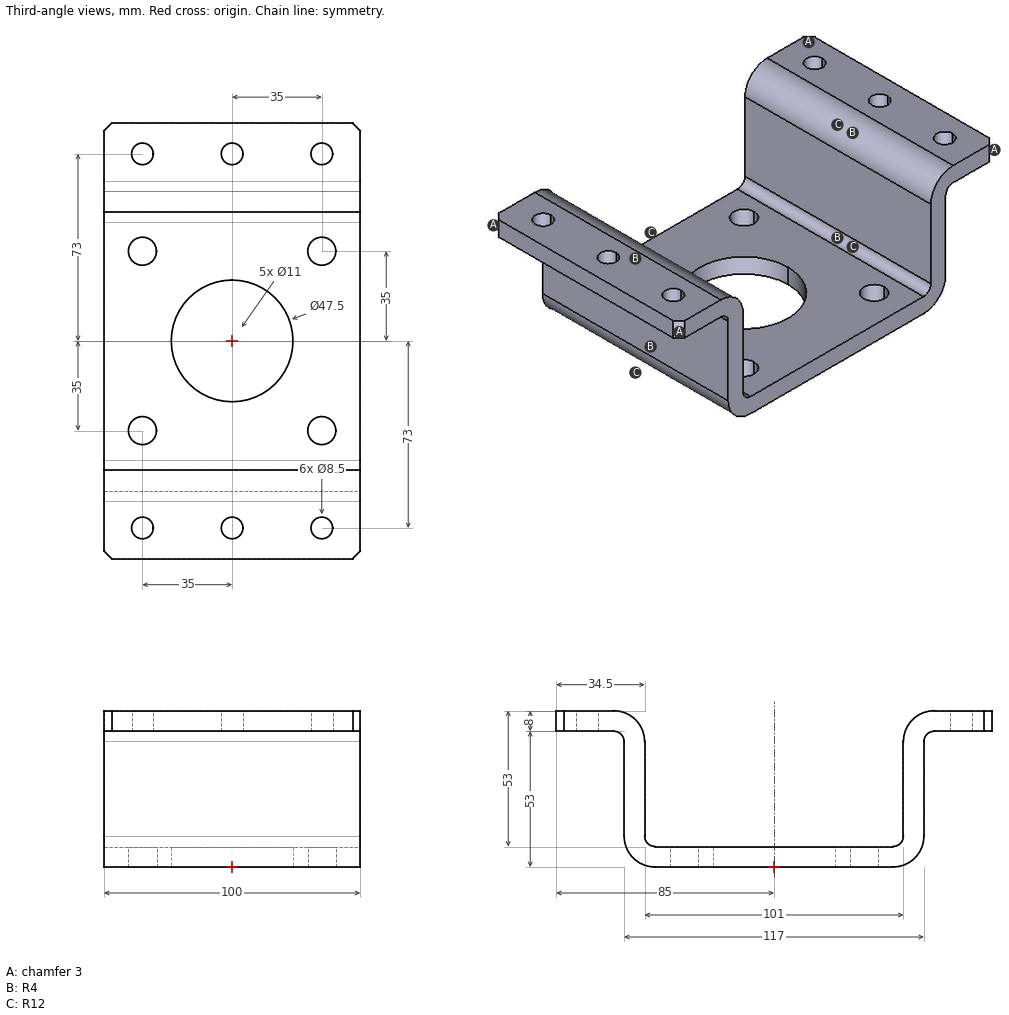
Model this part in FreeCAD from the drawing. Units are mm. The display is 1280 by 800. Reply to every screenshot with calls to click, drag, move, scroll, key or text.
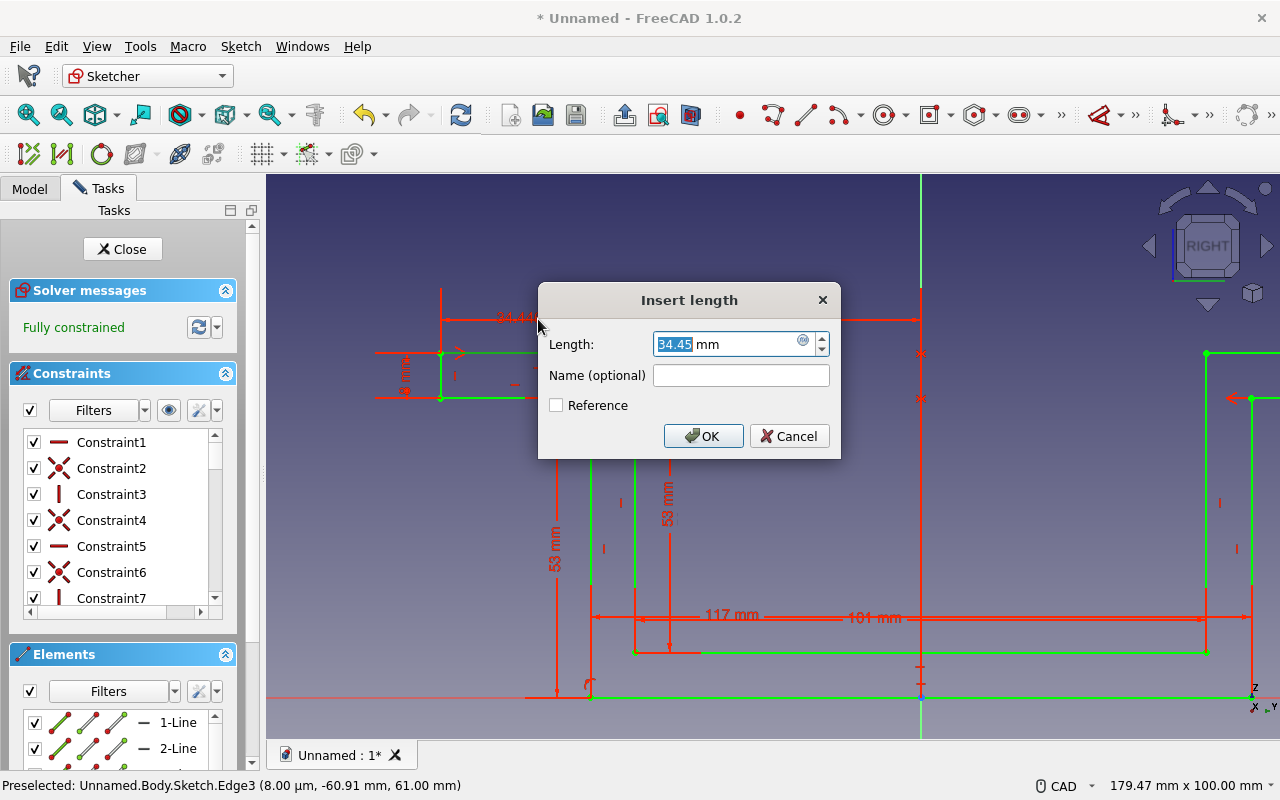
text(34.5)
key(Return)
key(Escape)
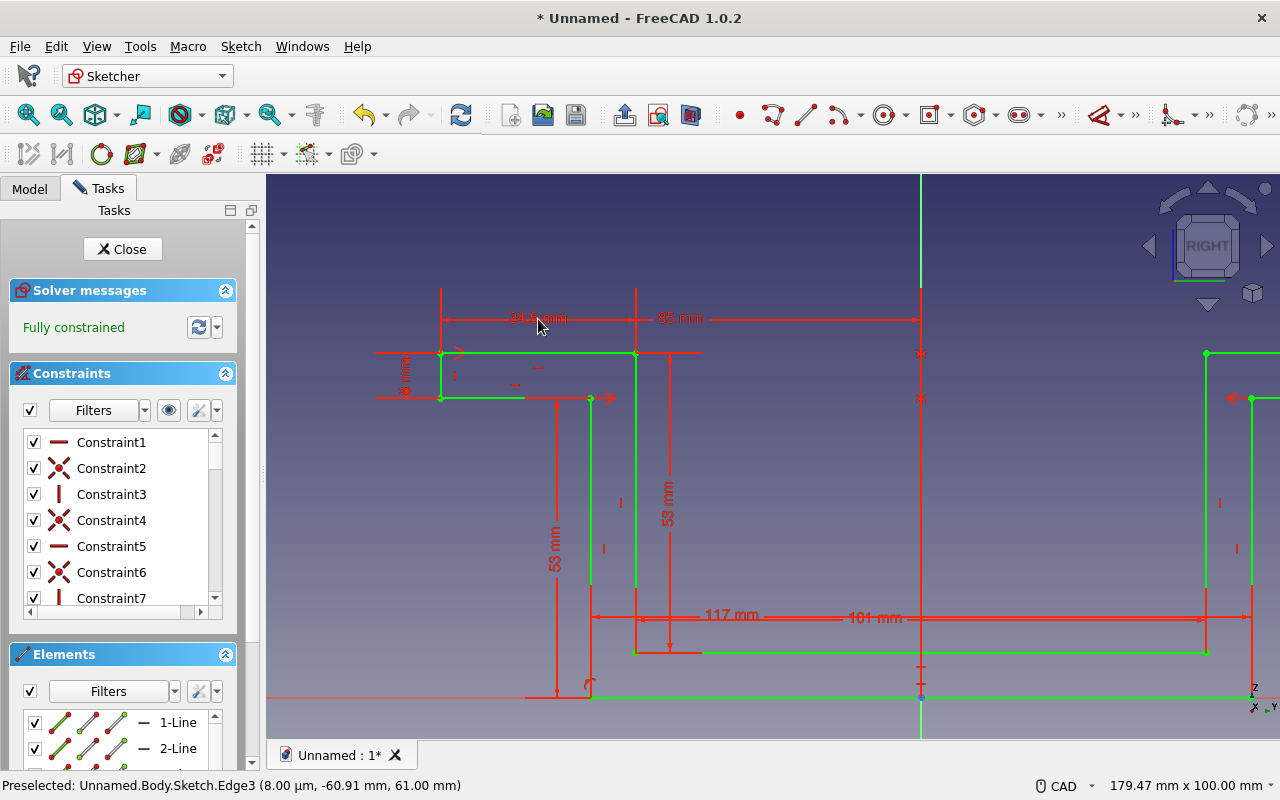
click(123, 249)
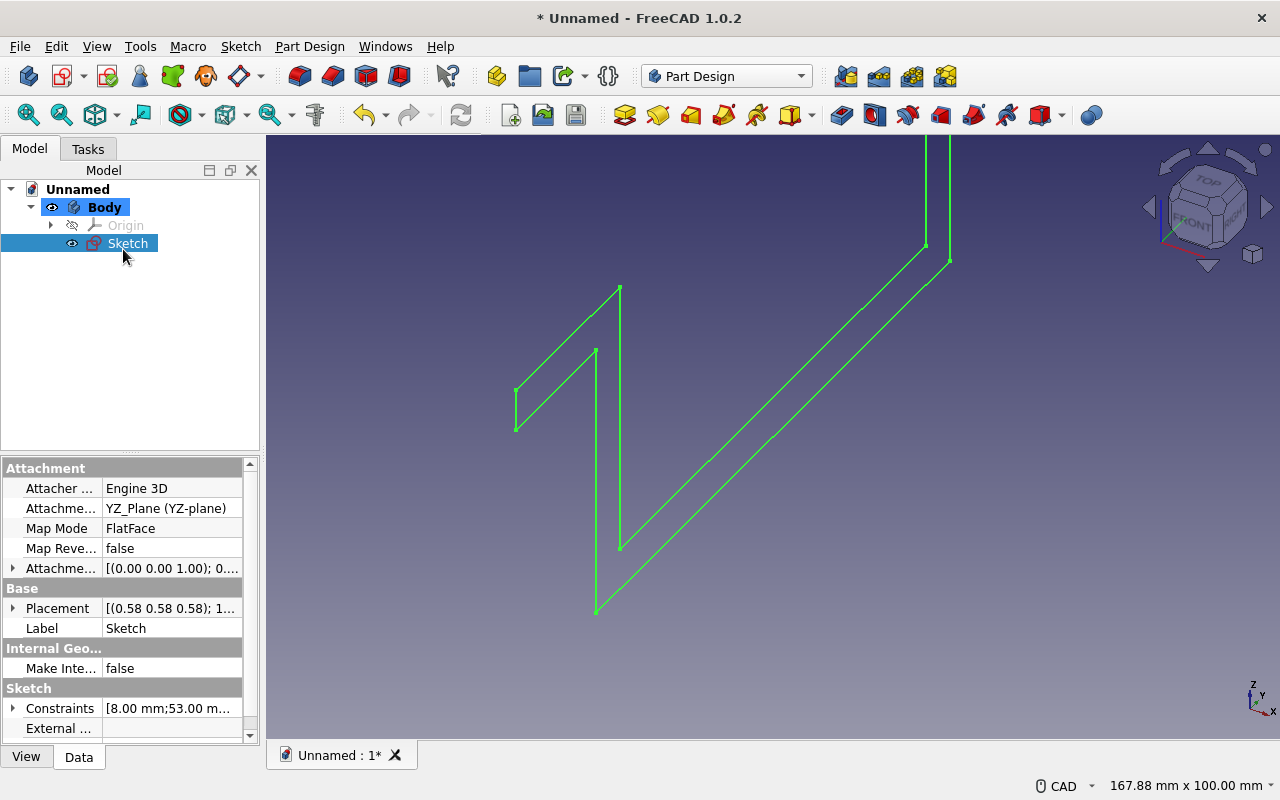
click(625, 116)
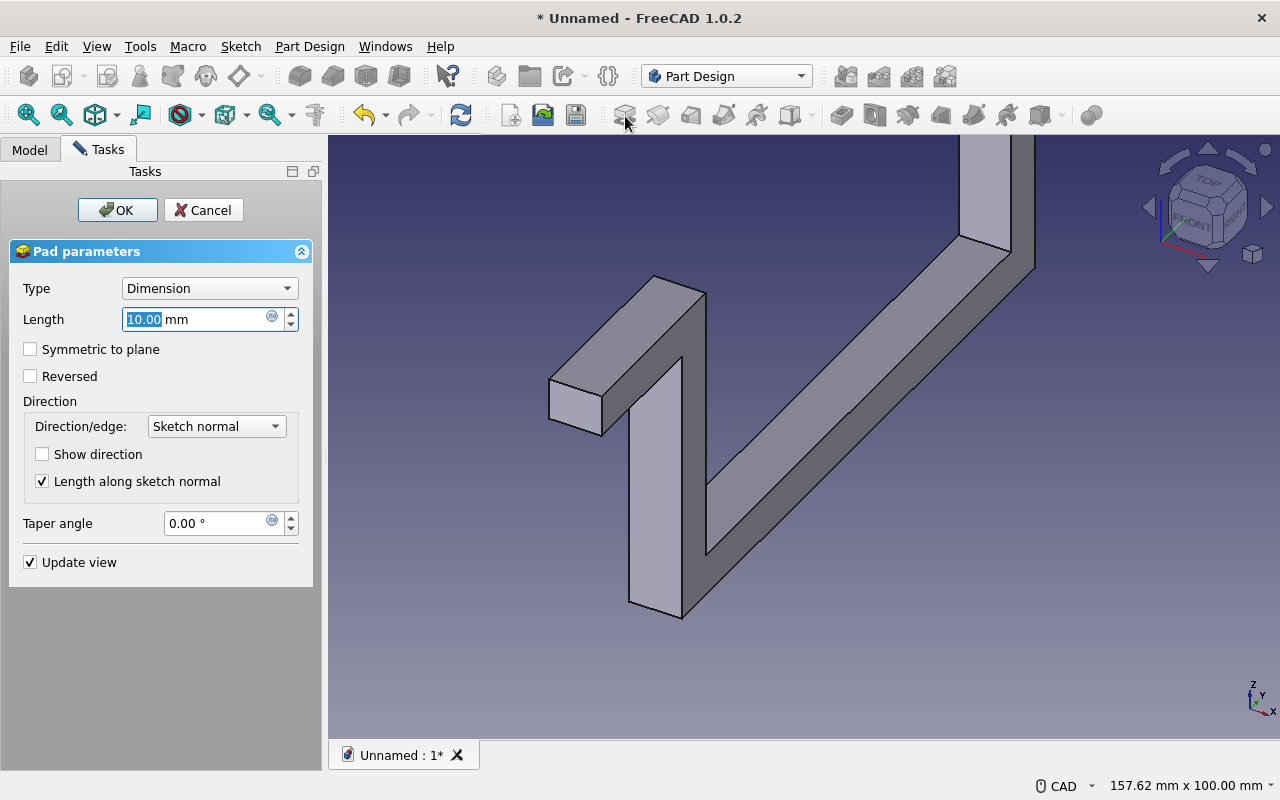
text(100)
key(Tab)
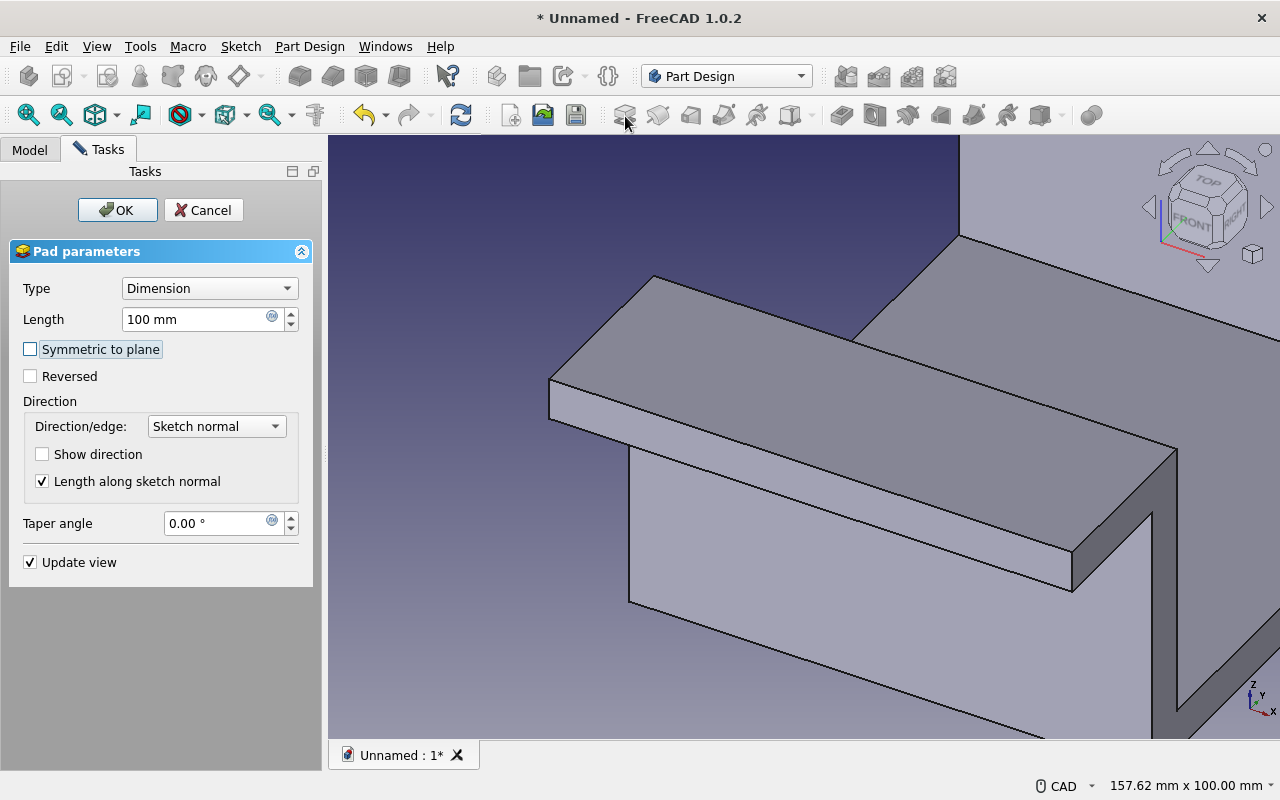
click(31, 349)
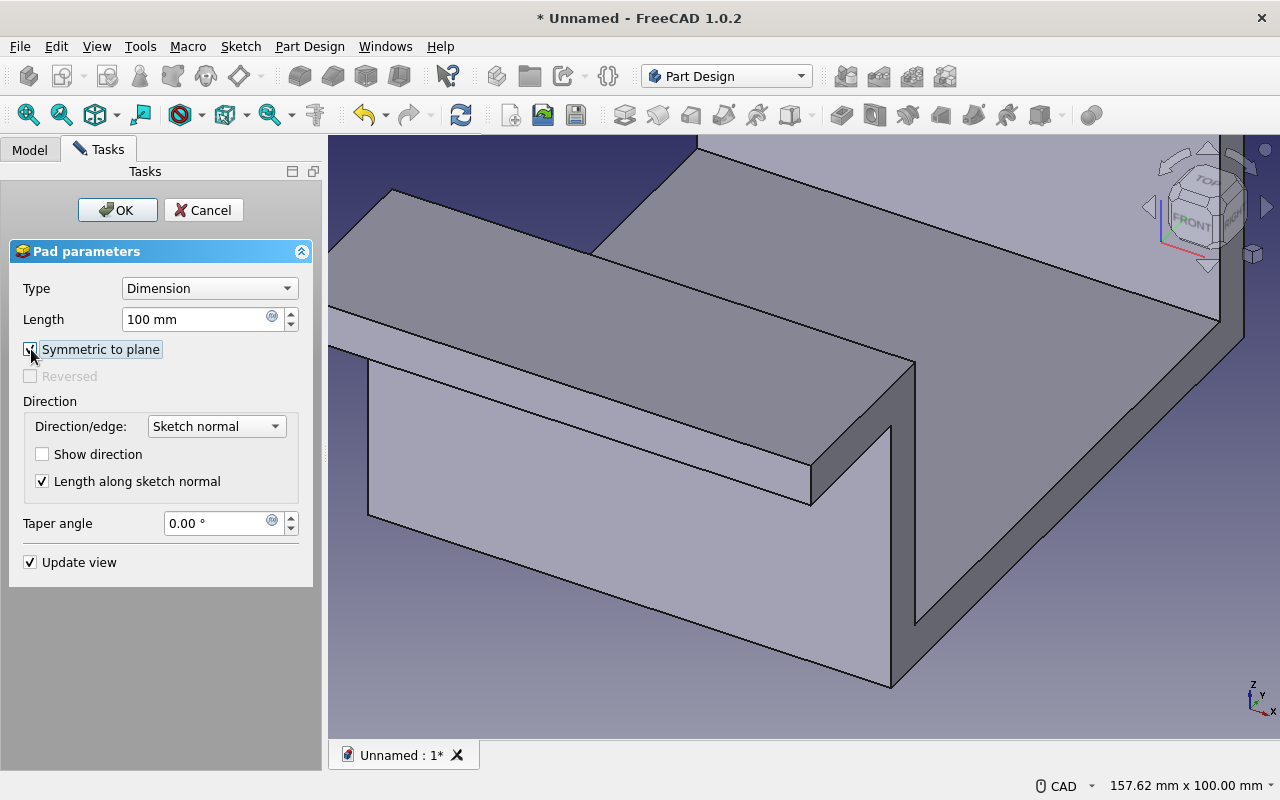
click(118, 210)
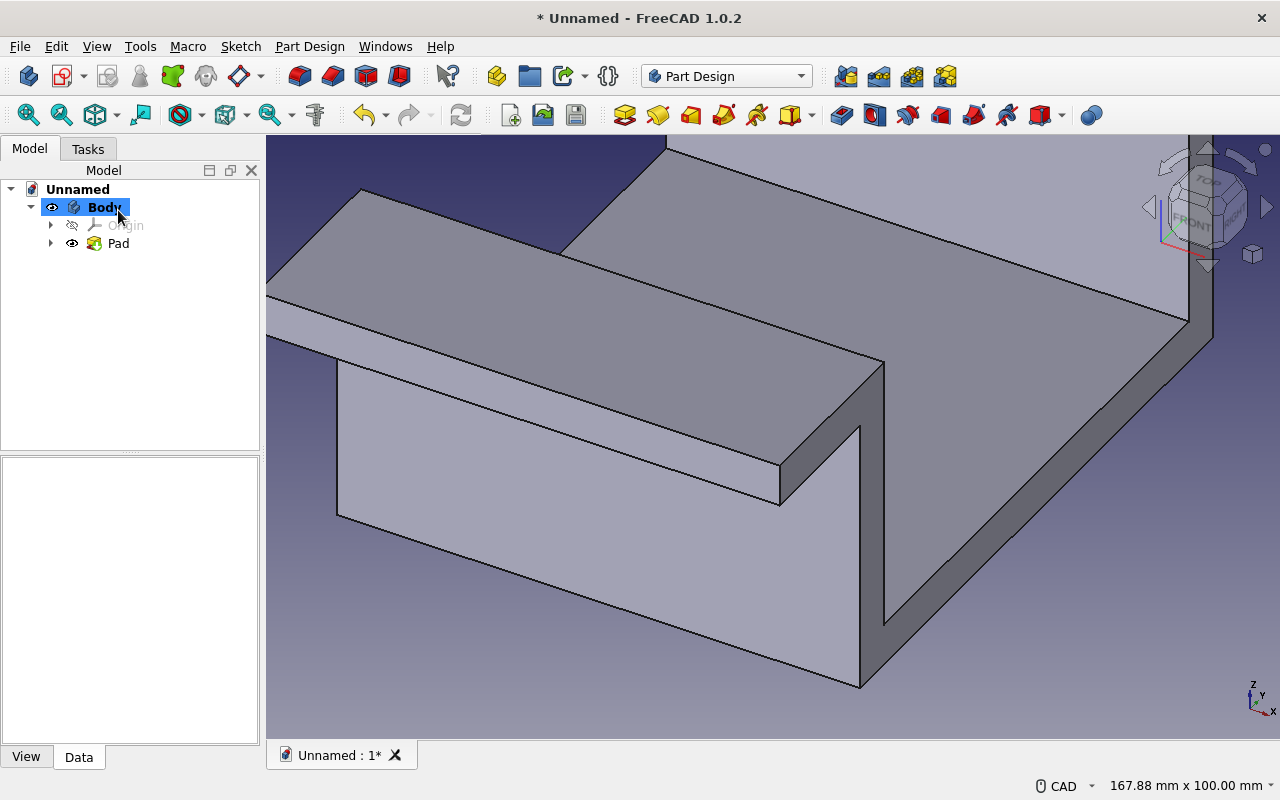
key(v)
key(f)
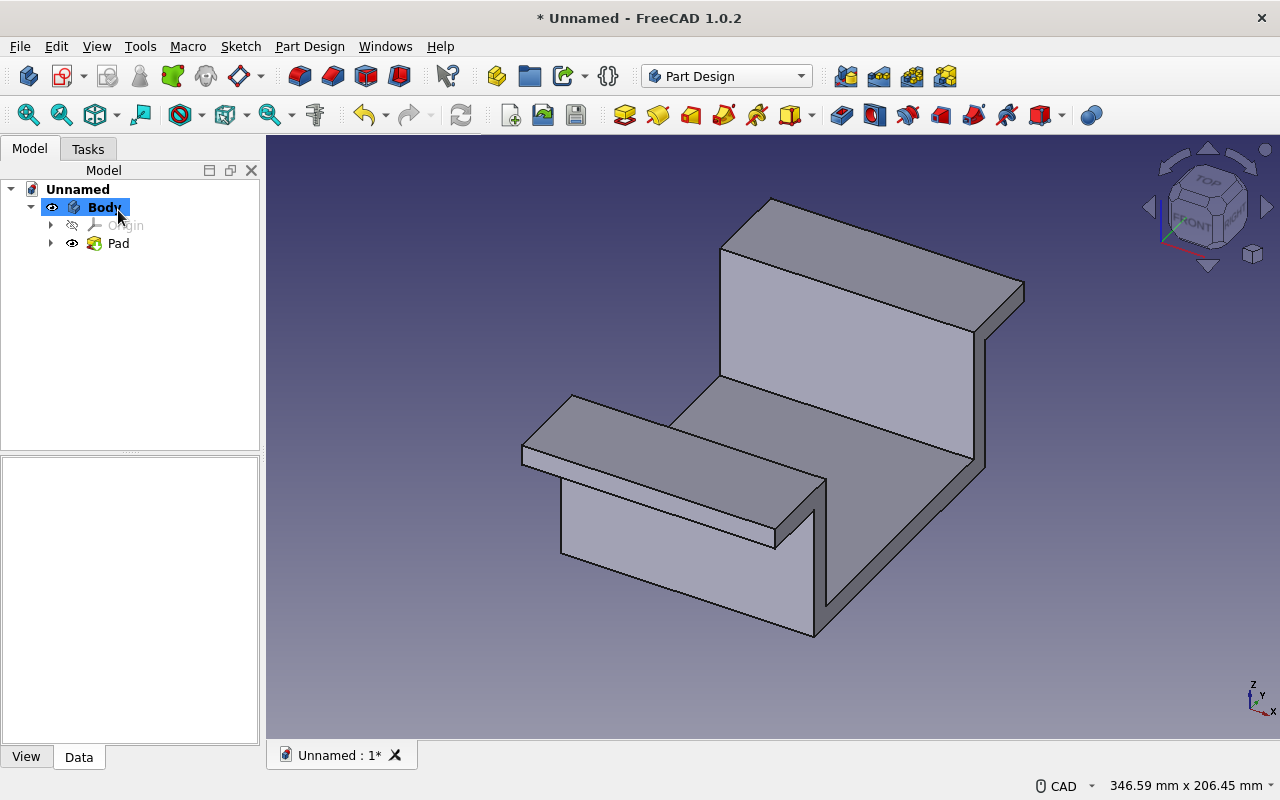
key(5)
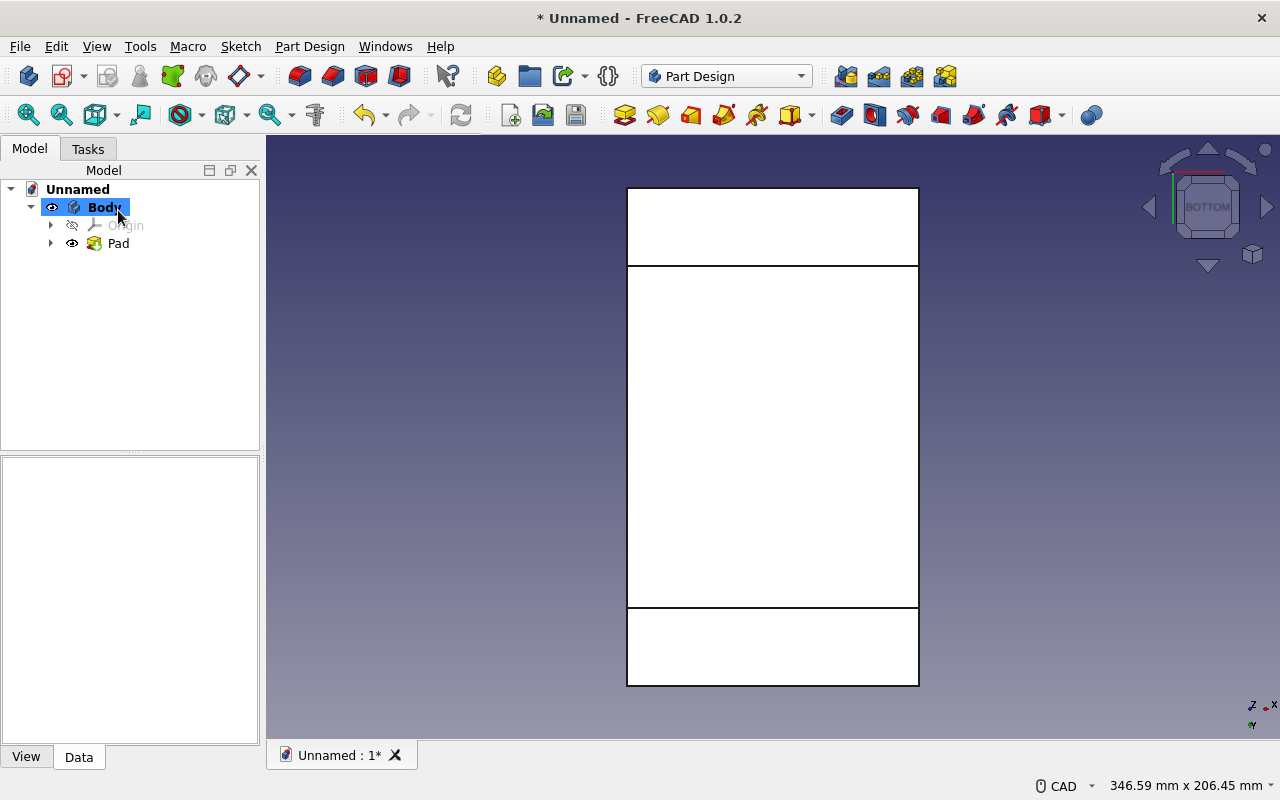
click(773, 436)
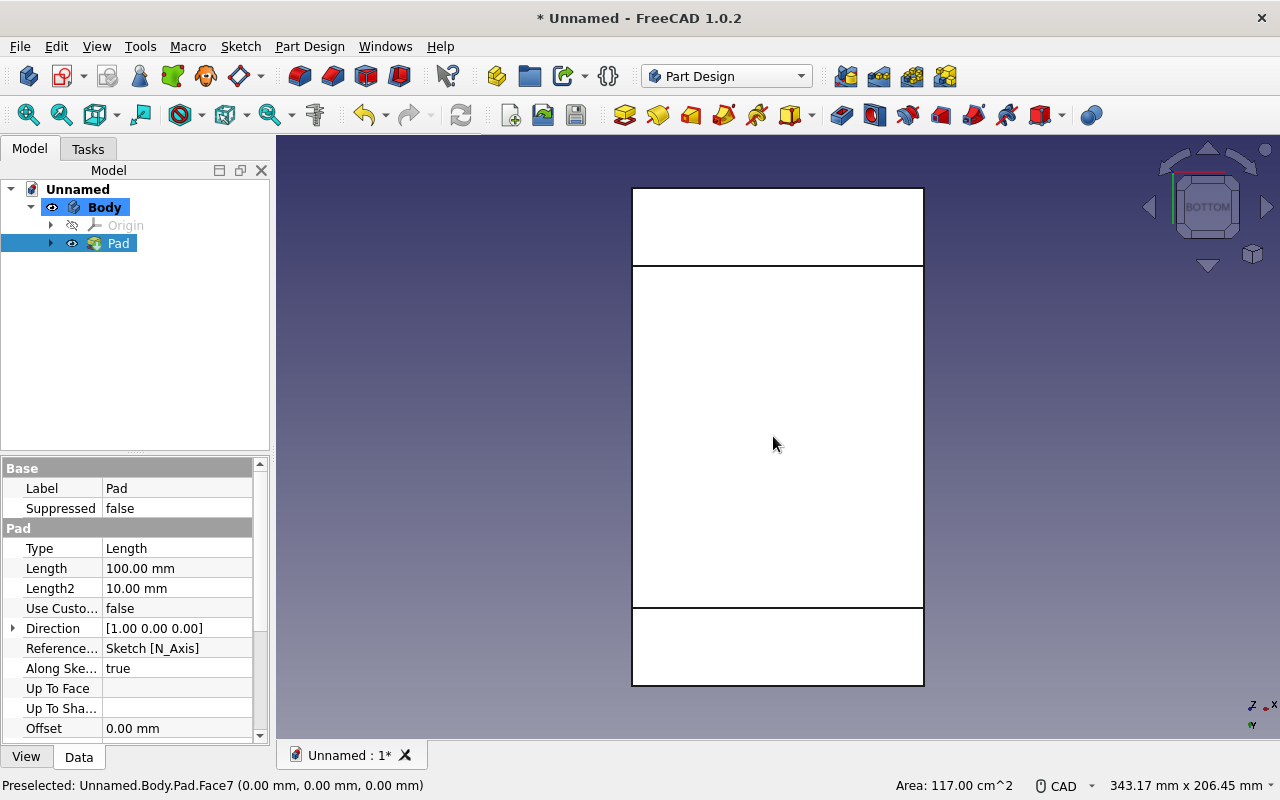
click(62, 76)